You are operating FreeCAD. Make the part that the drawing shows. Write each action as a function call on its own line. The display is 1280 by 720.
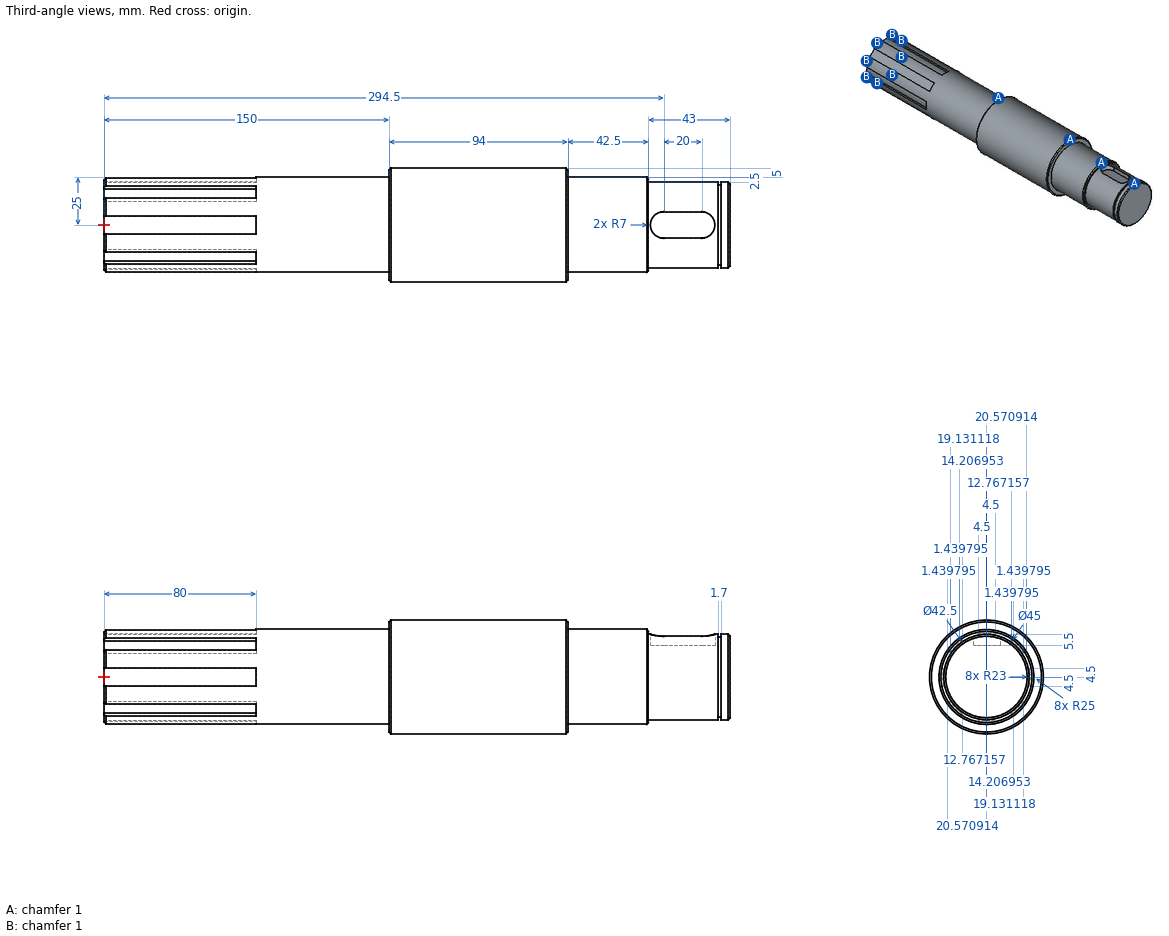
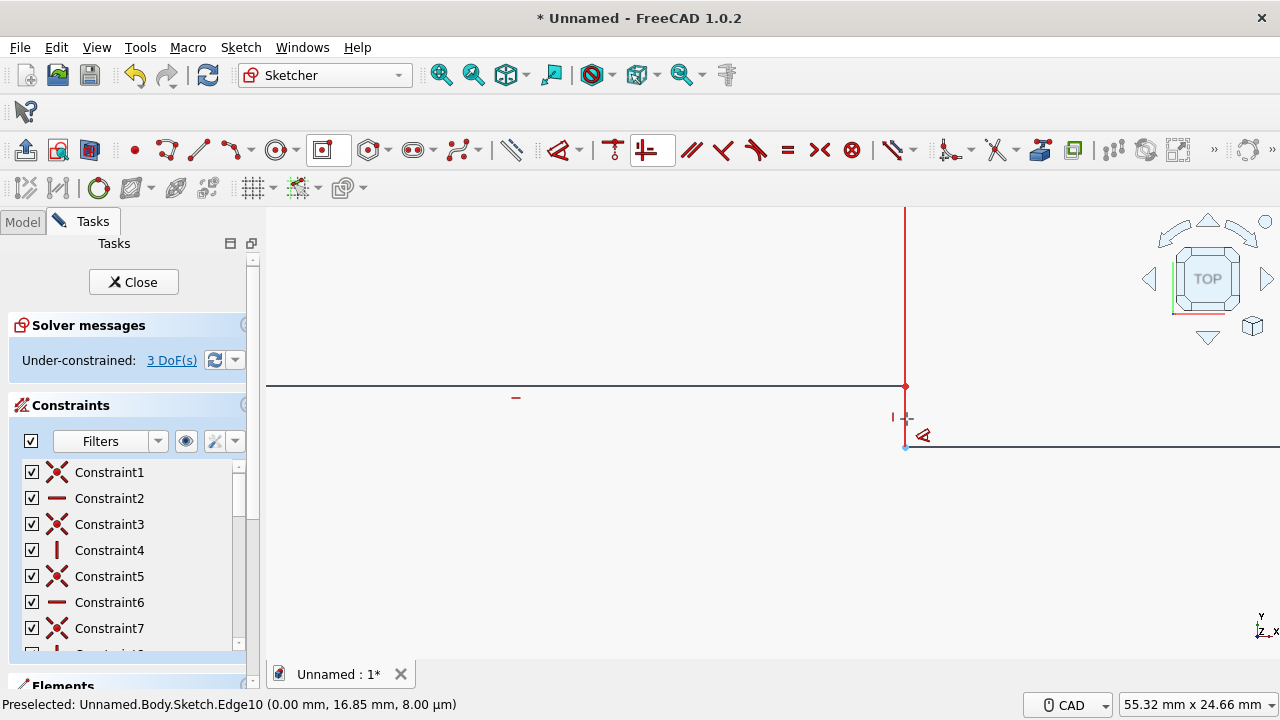
click(905, 417)
click(939, 417)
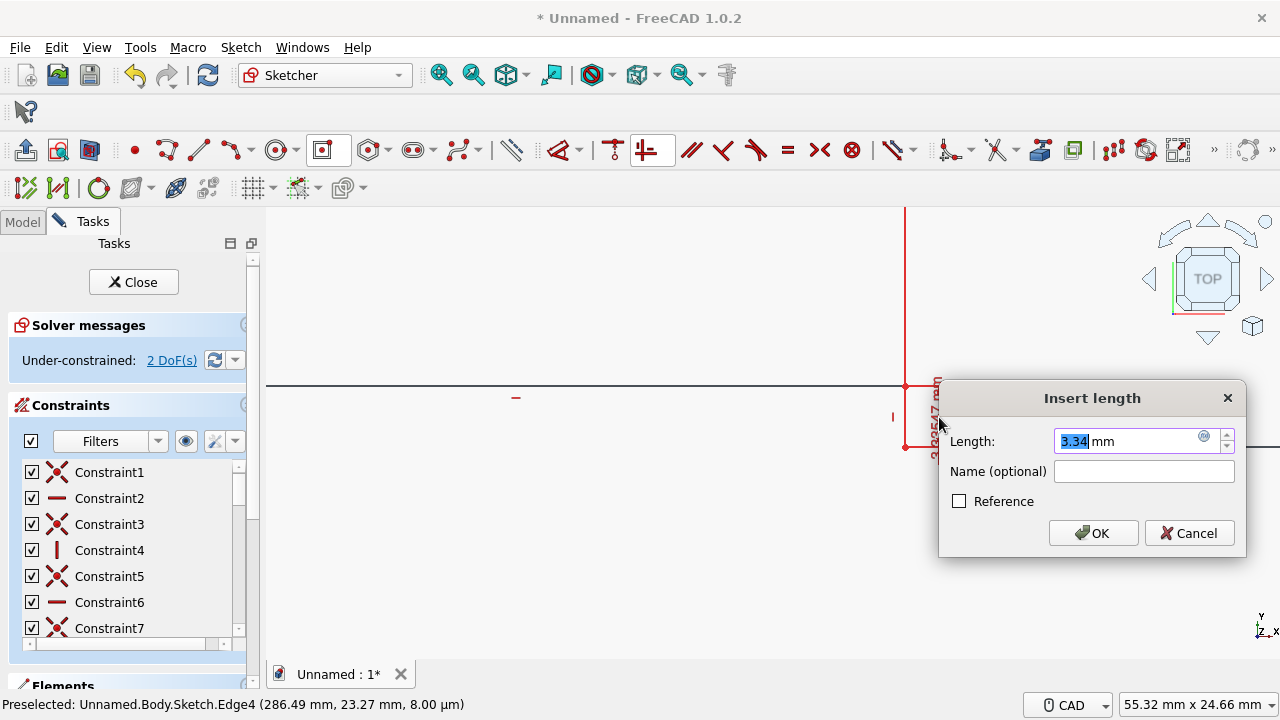
text(2.5)
key(Return)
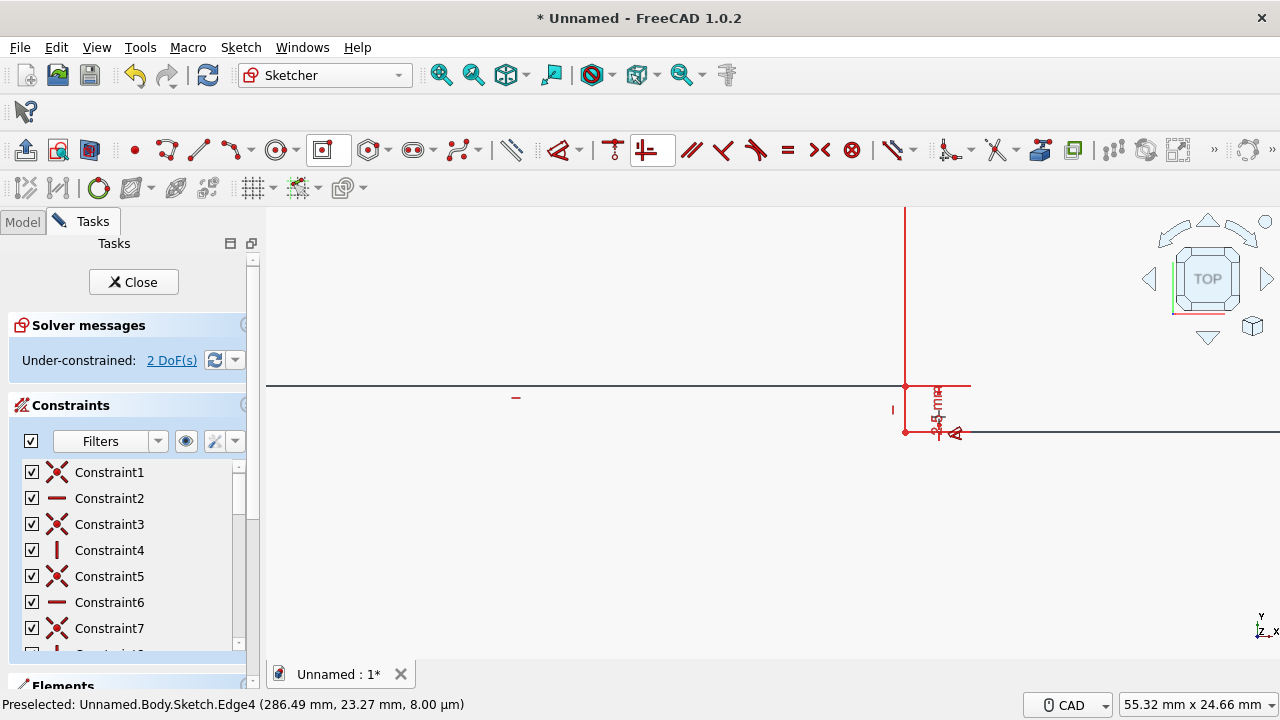
scroll(907, 419, down, 12)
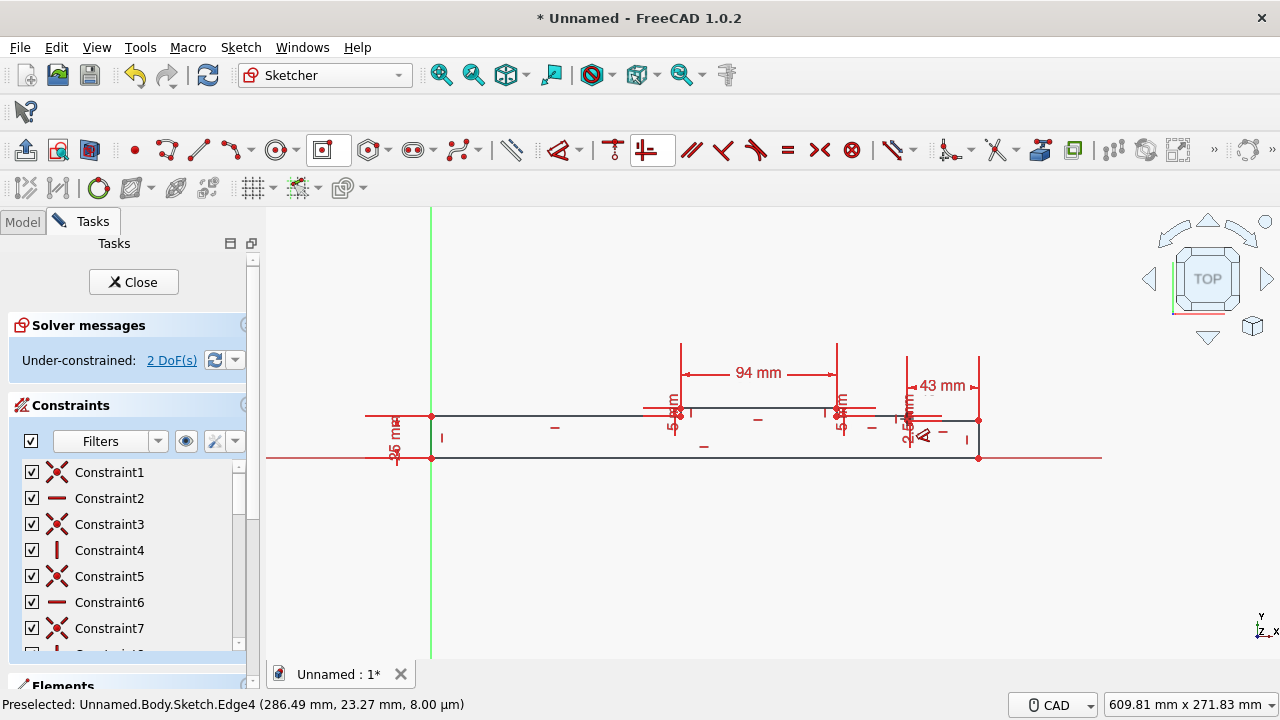
click(606, 416)
click(556, 382)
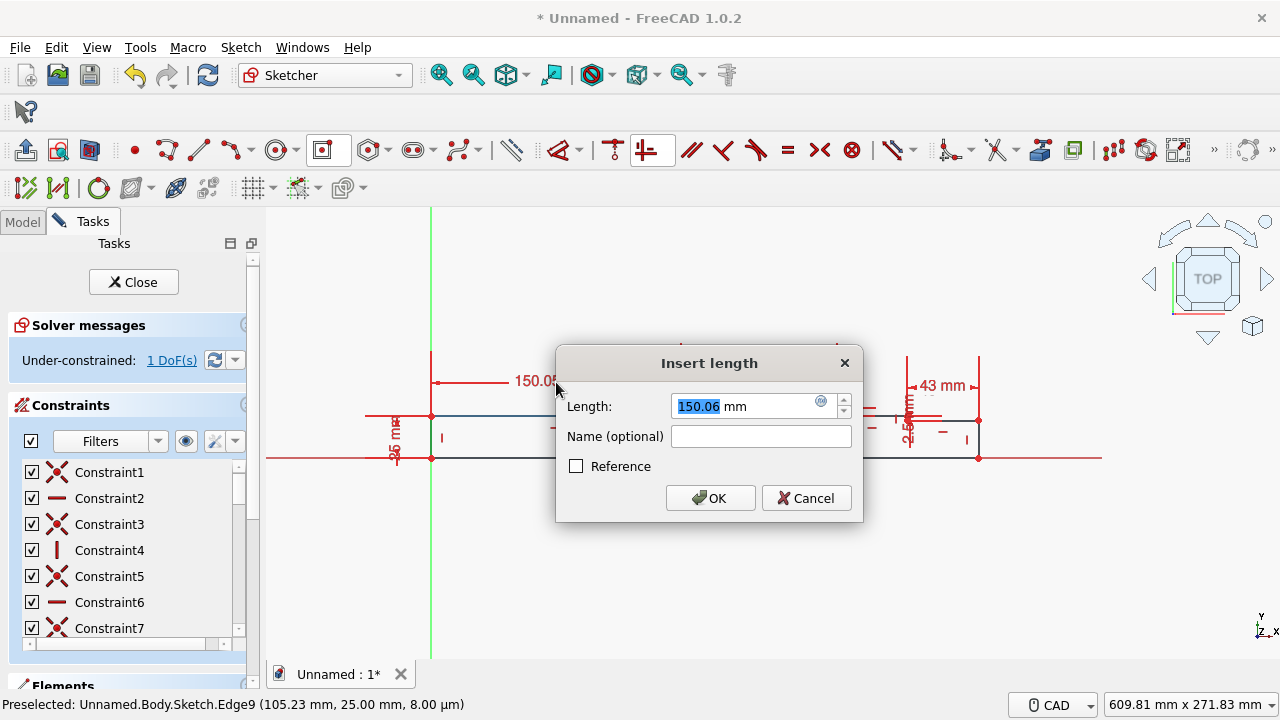
text(150)
key(Return)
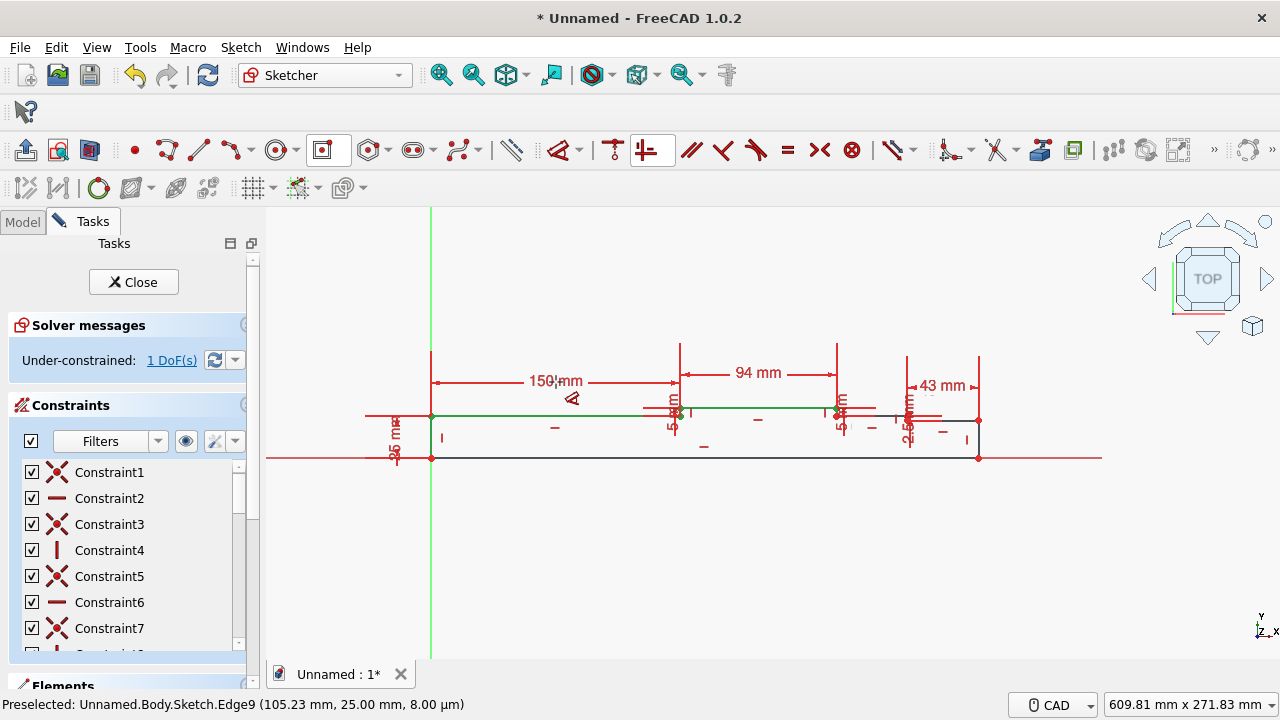
click(886, 416)
click(872, 382)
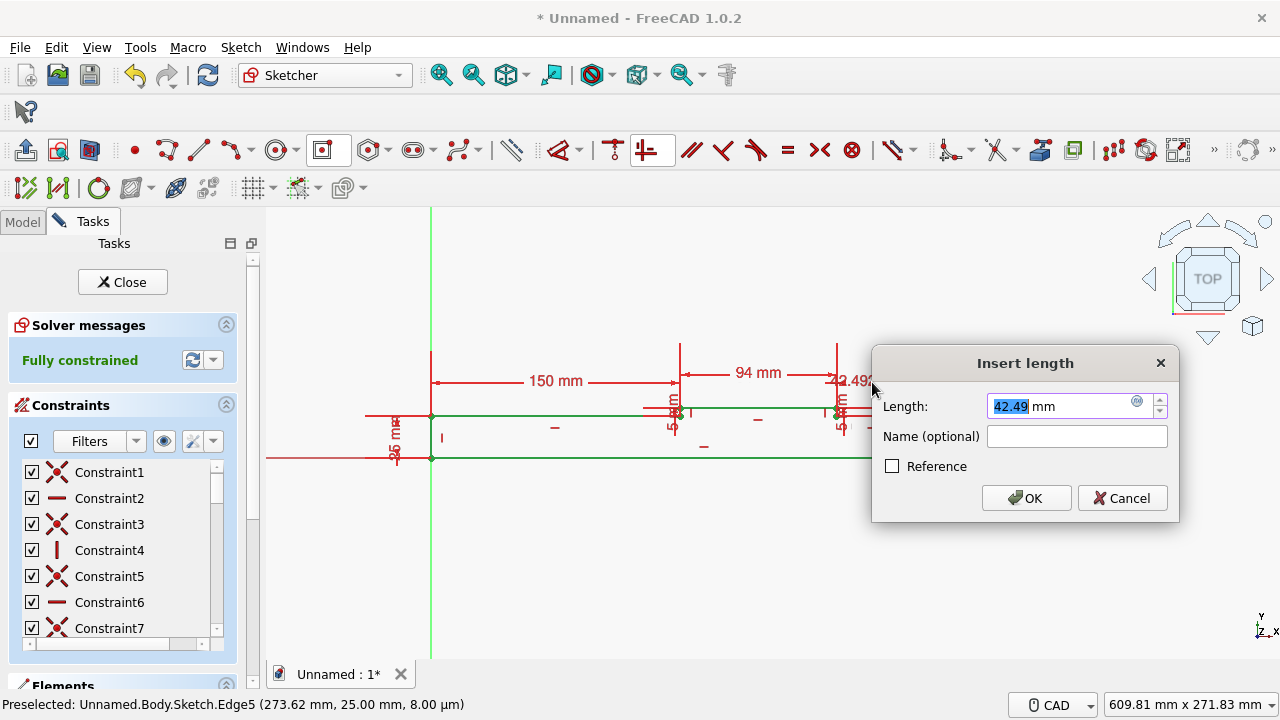
text(42.5)
key(Return)
key(Escape)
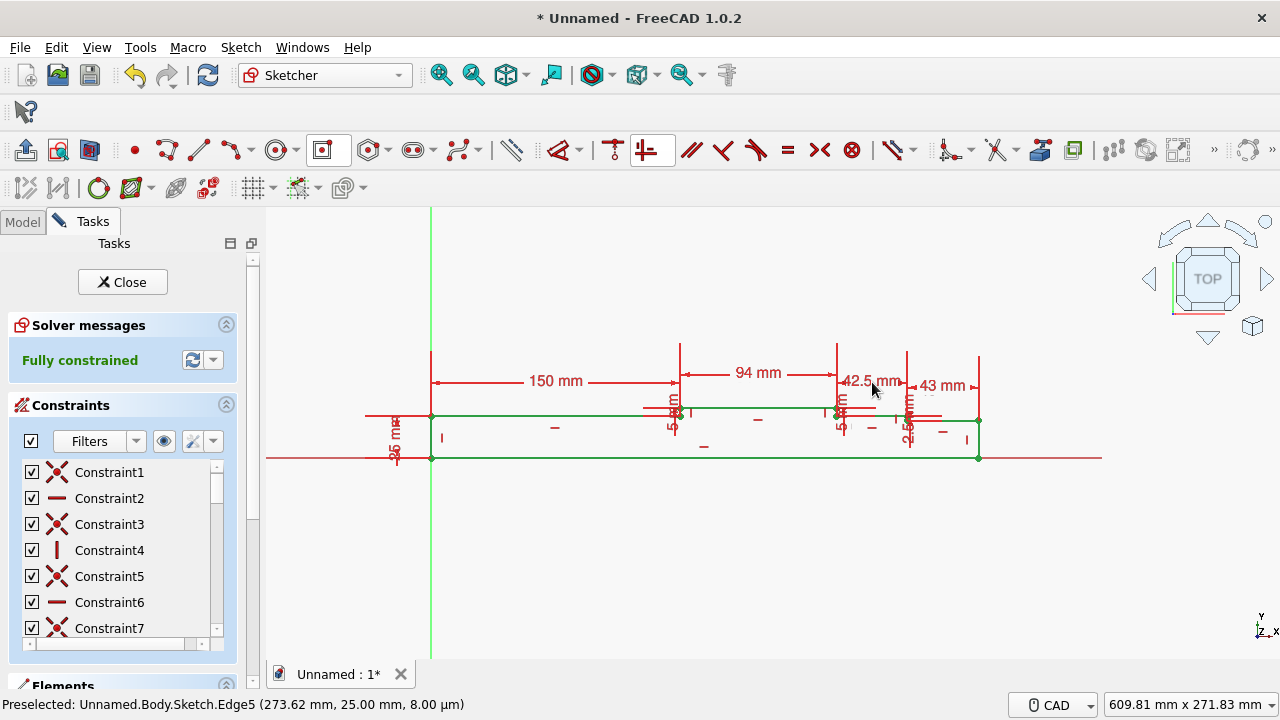
click(123, 282)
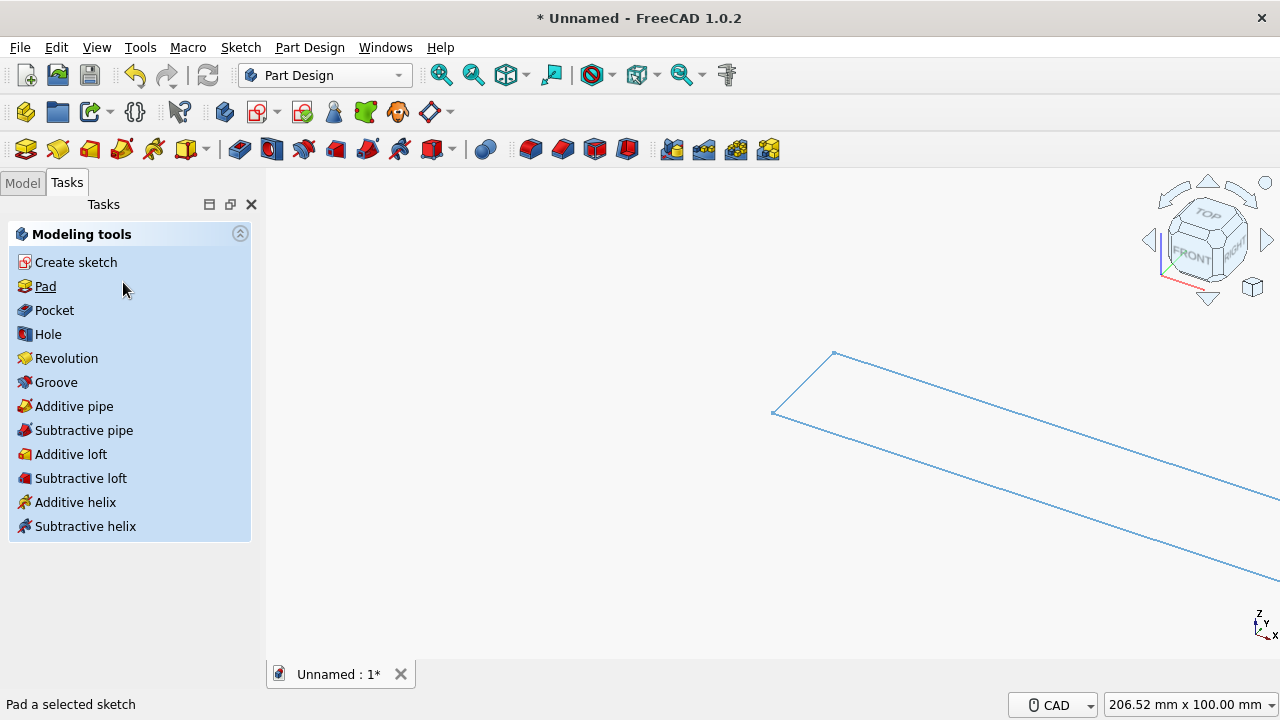
click(58, 150)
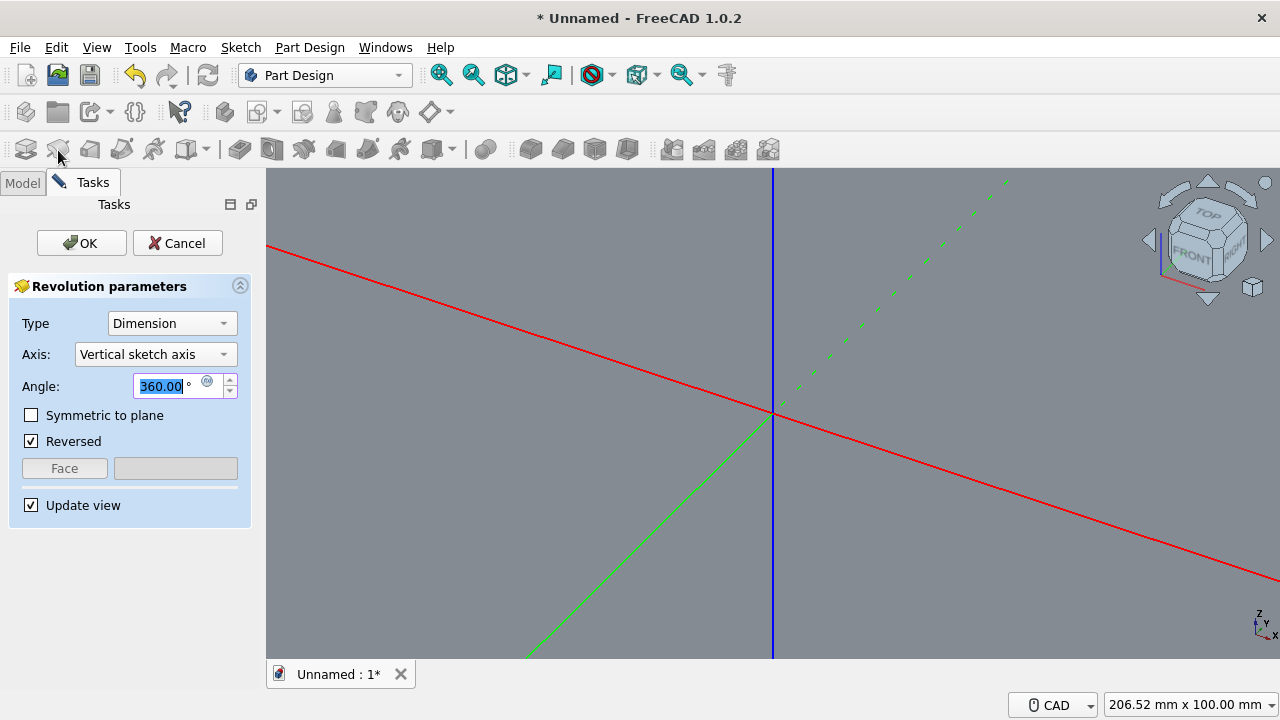
click(156, 354)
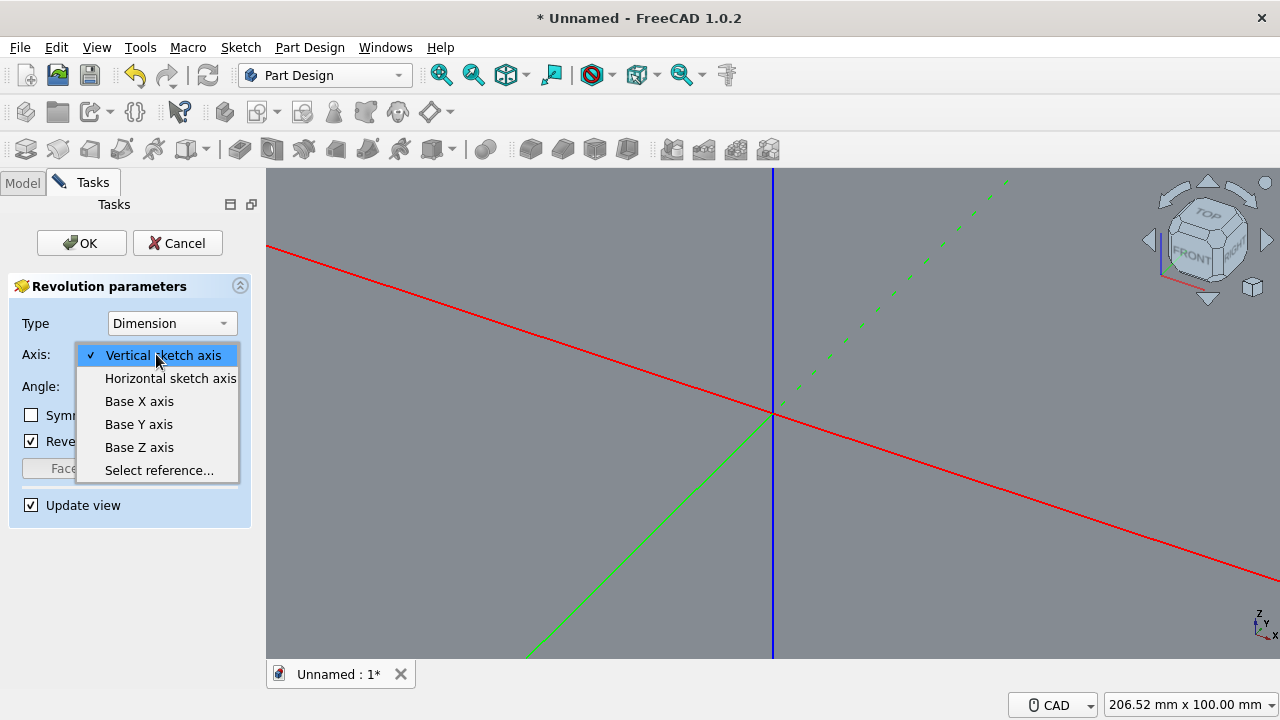
click(156, 378)